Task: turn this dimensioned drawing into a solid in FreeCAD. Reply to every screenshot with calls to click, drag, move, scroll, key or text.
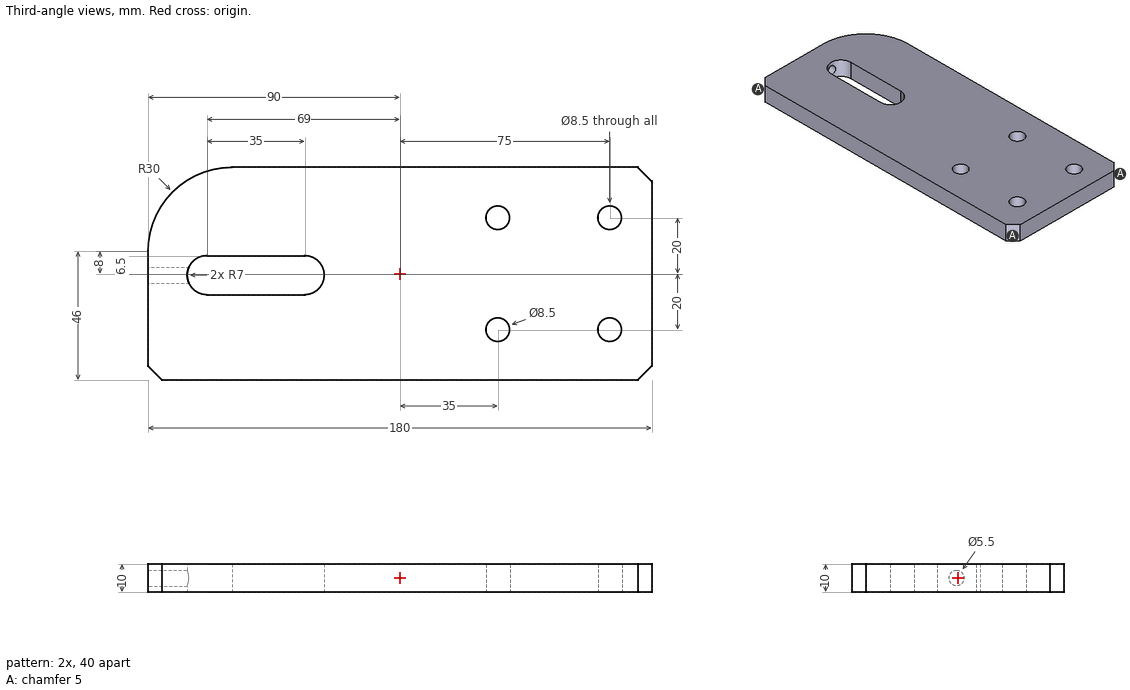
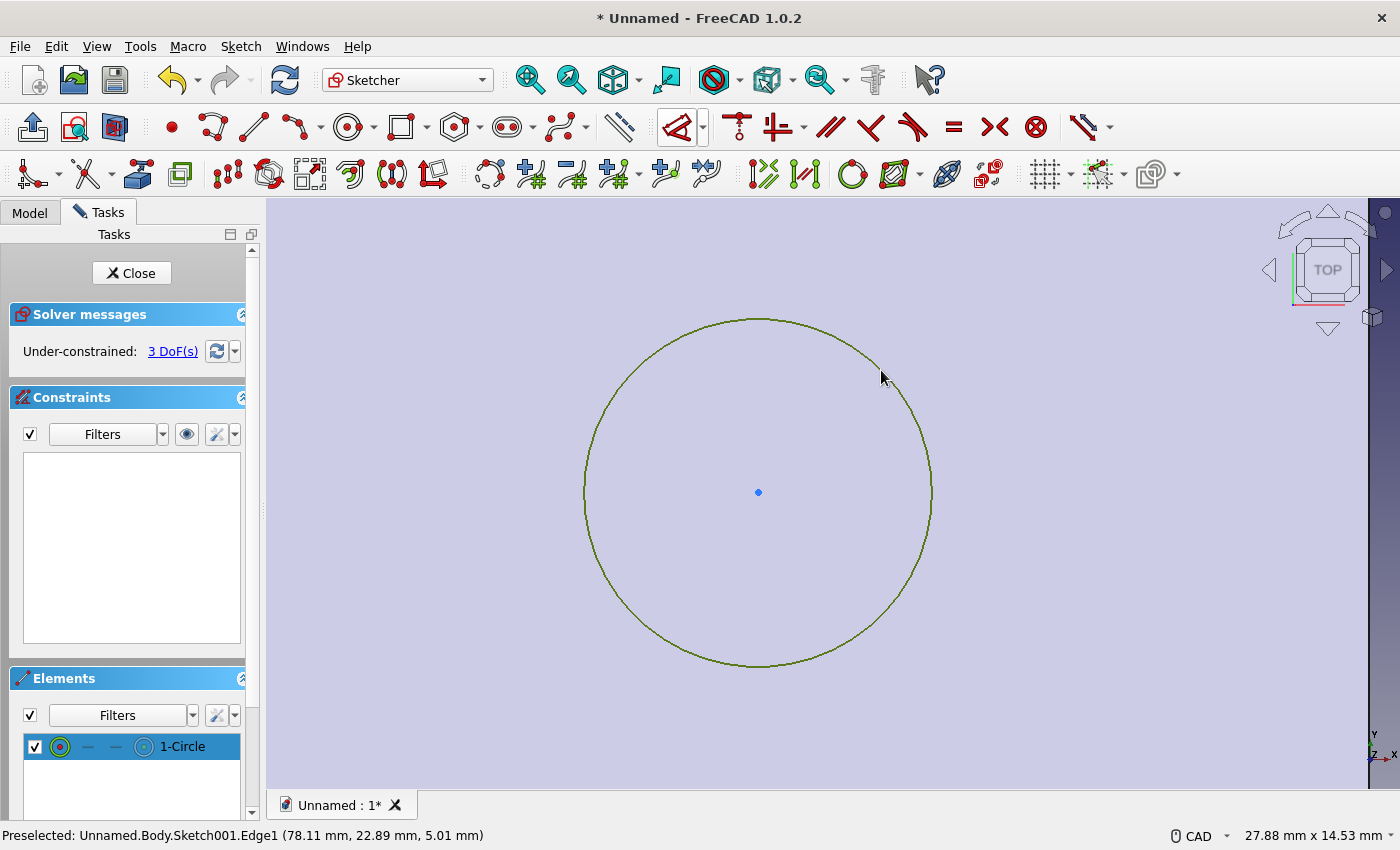
key(k)
key(o)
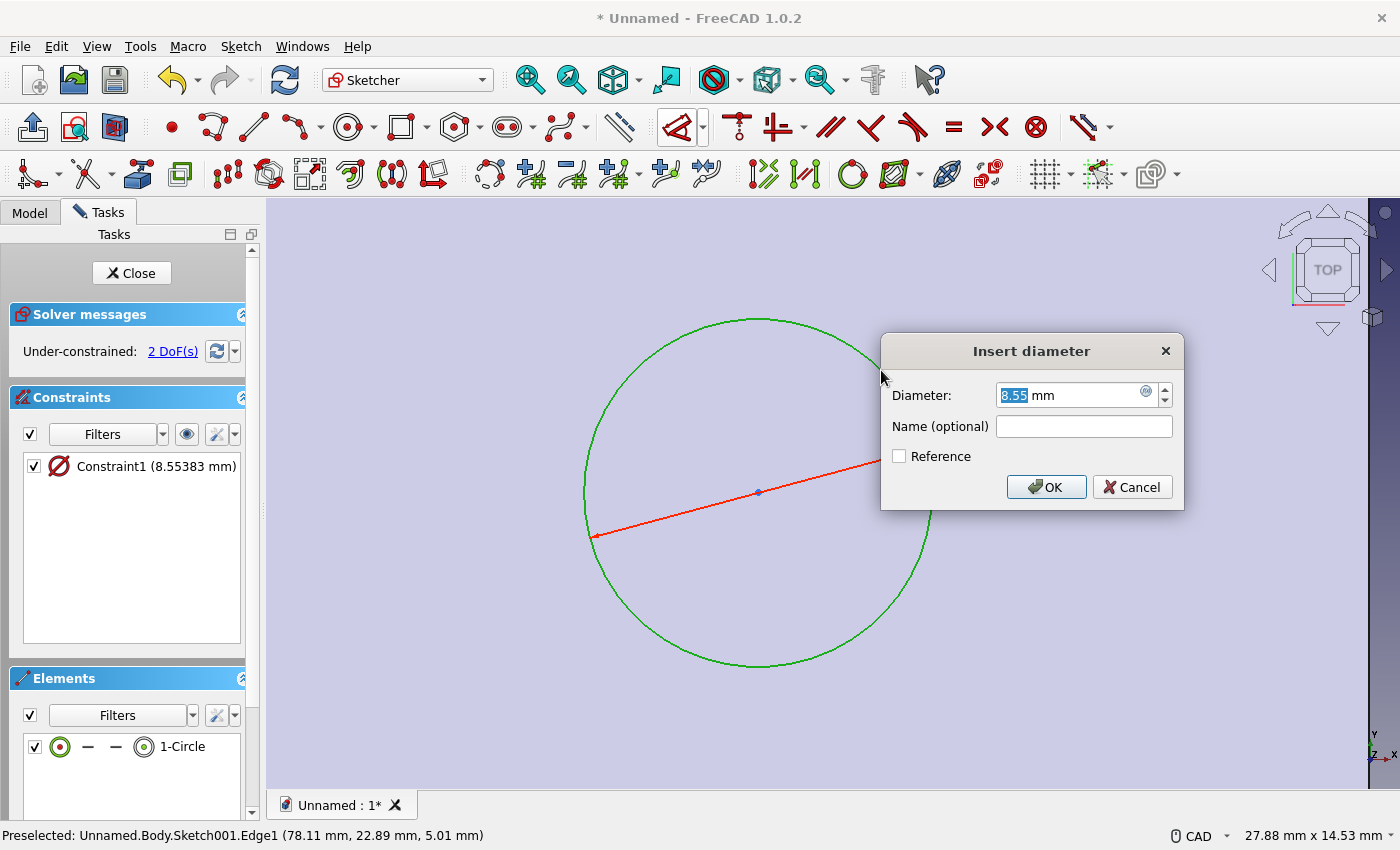
text(8.5)
key(Return)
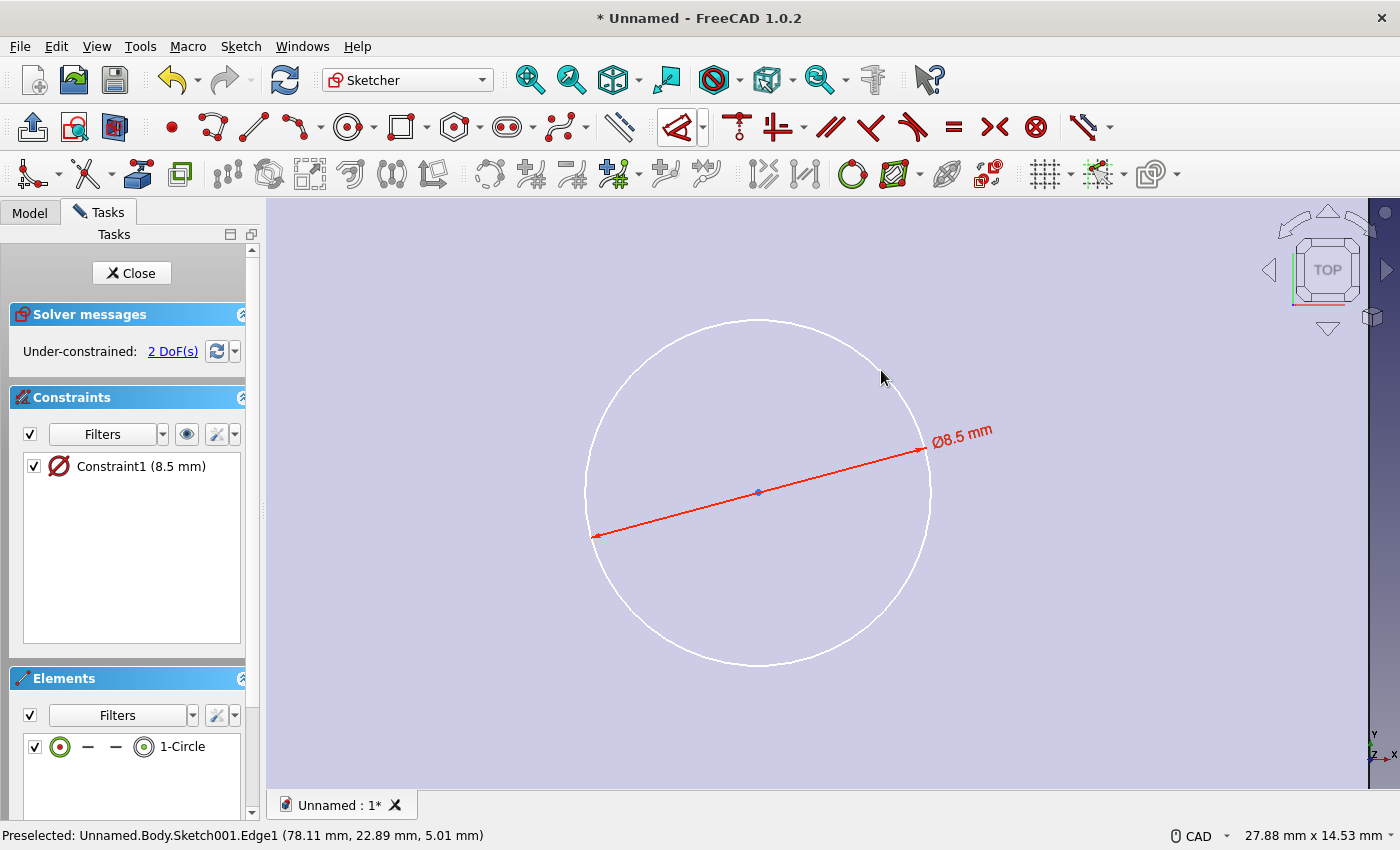
click(758, 493)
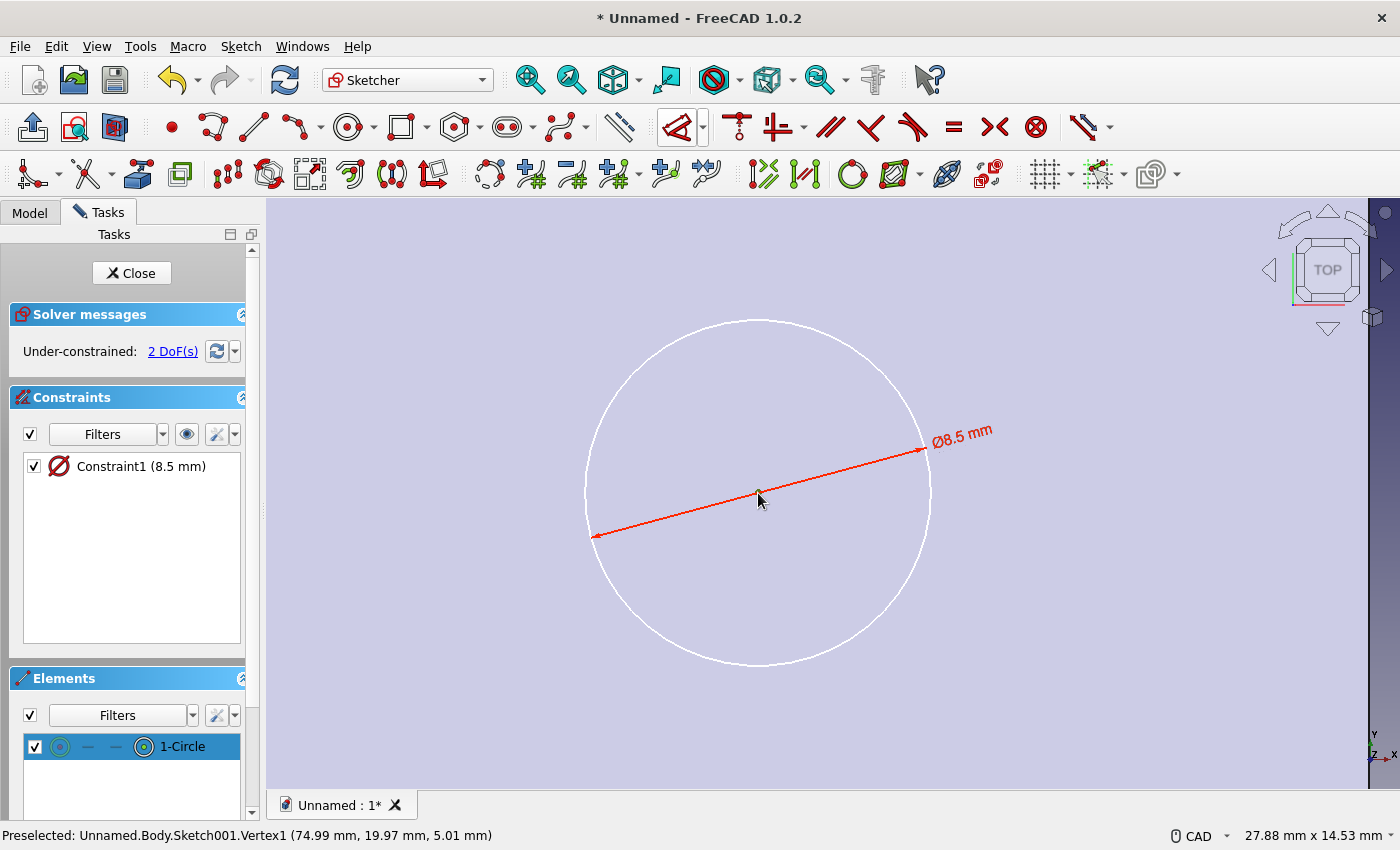
key(l)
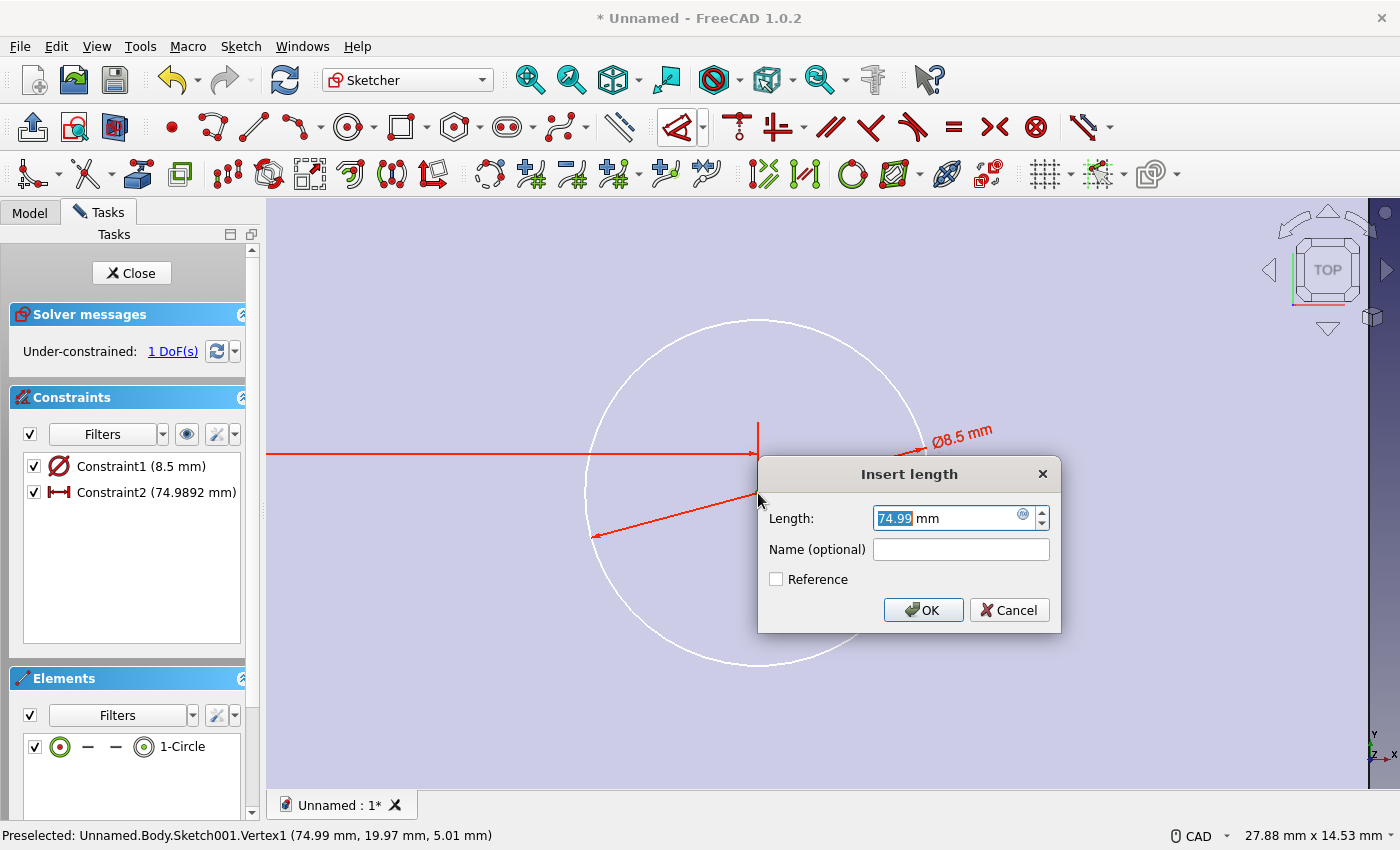
text(75)
key(Return)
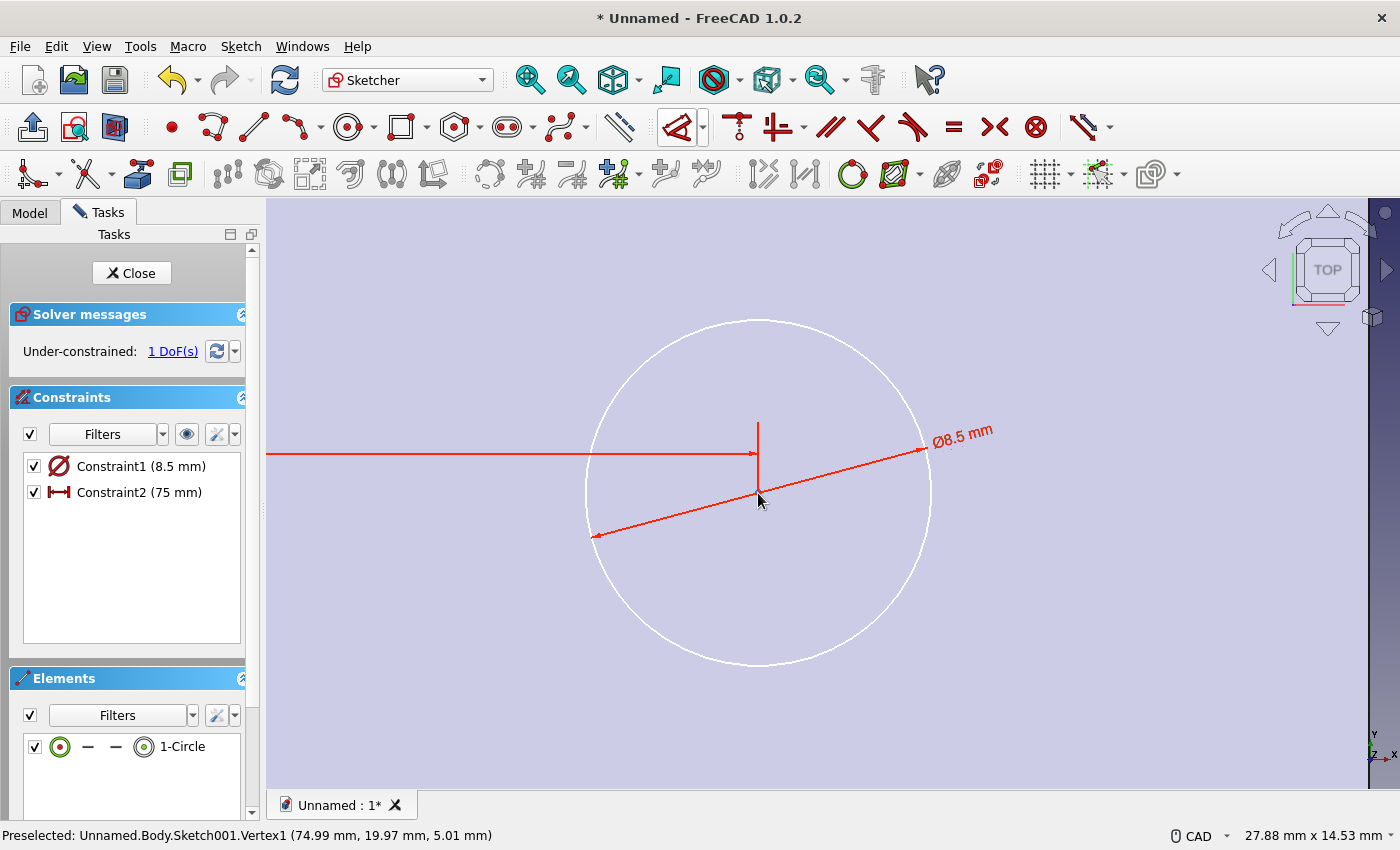
click(758, 493)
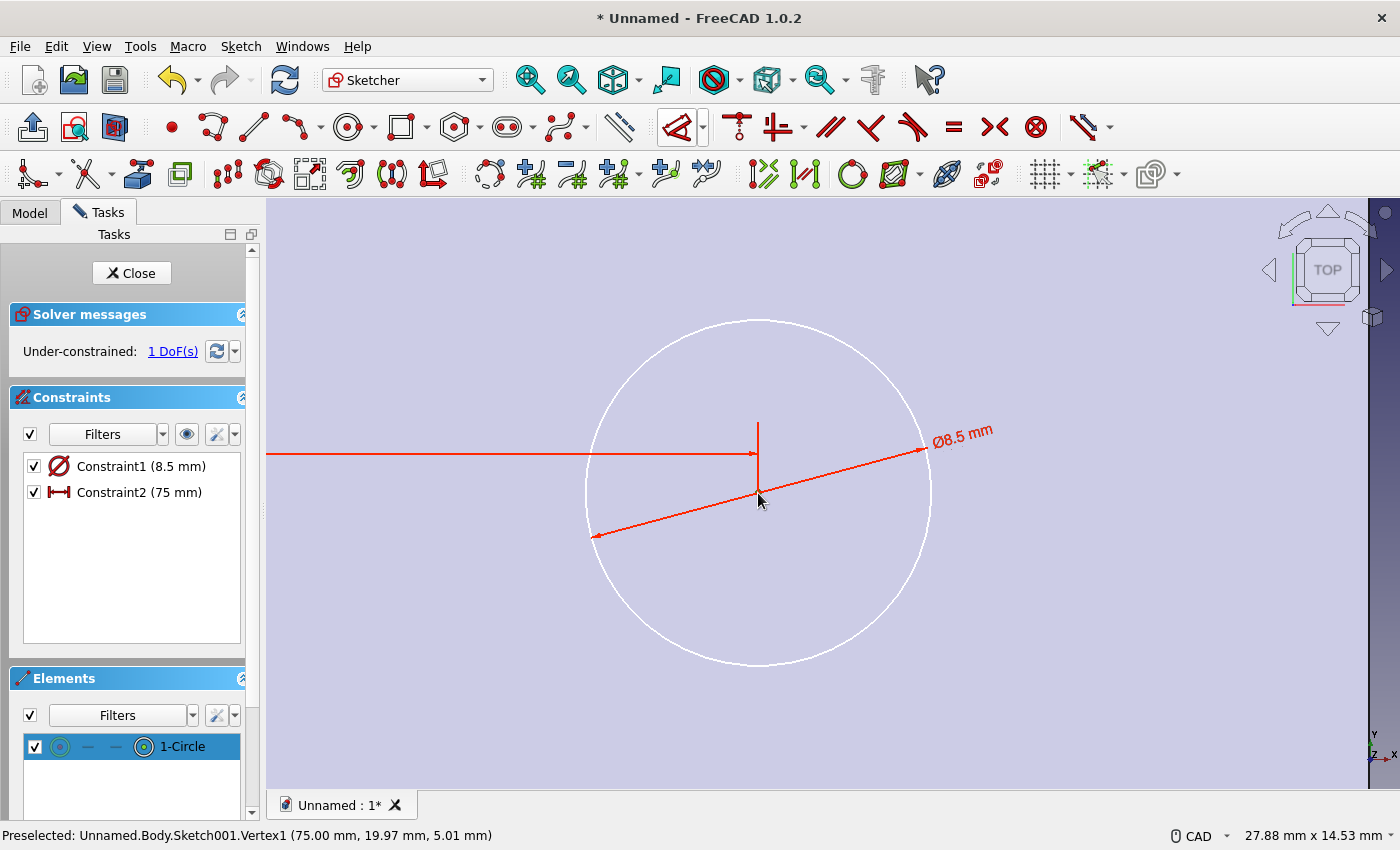
key(i)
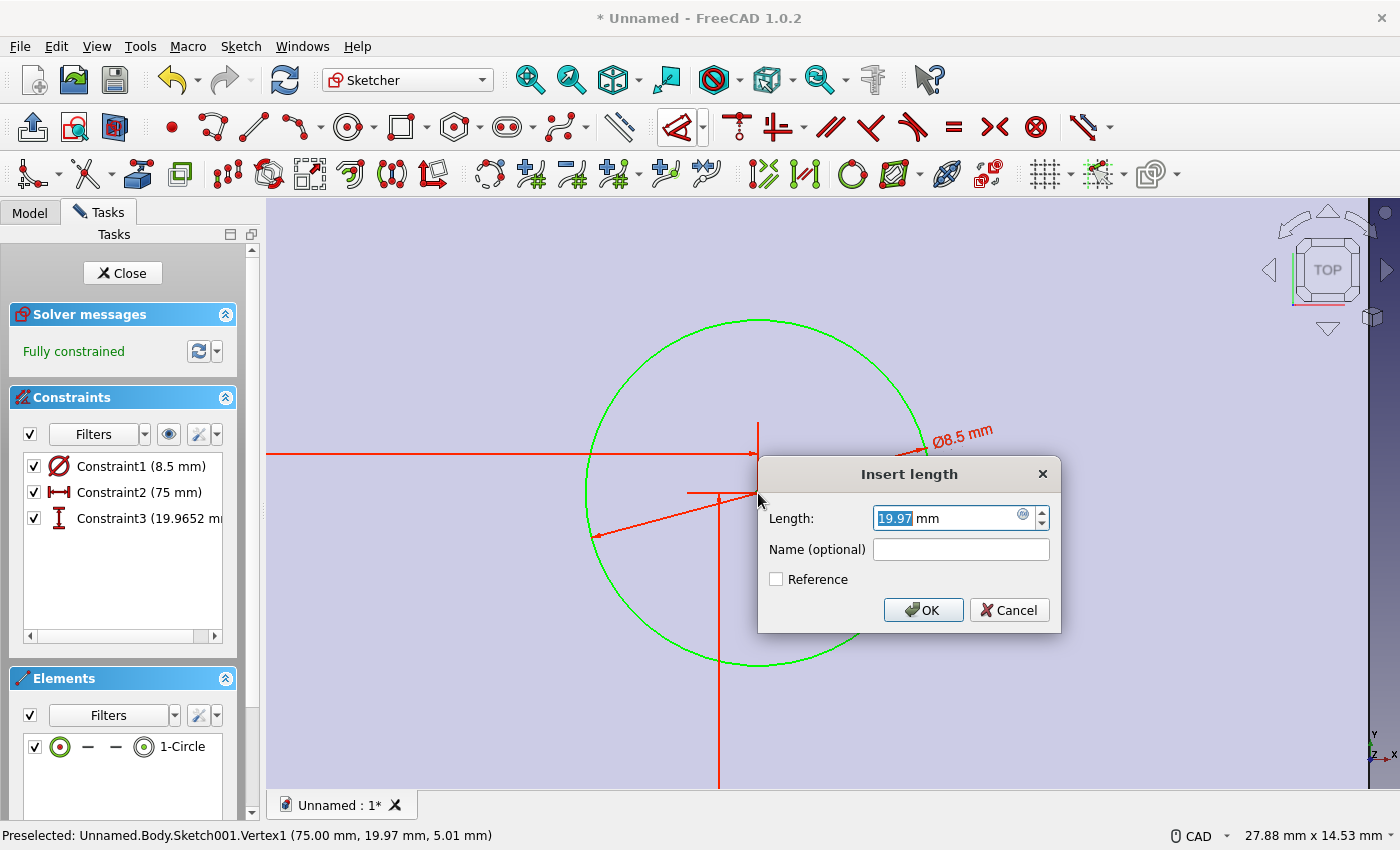
text(20)
key(Return)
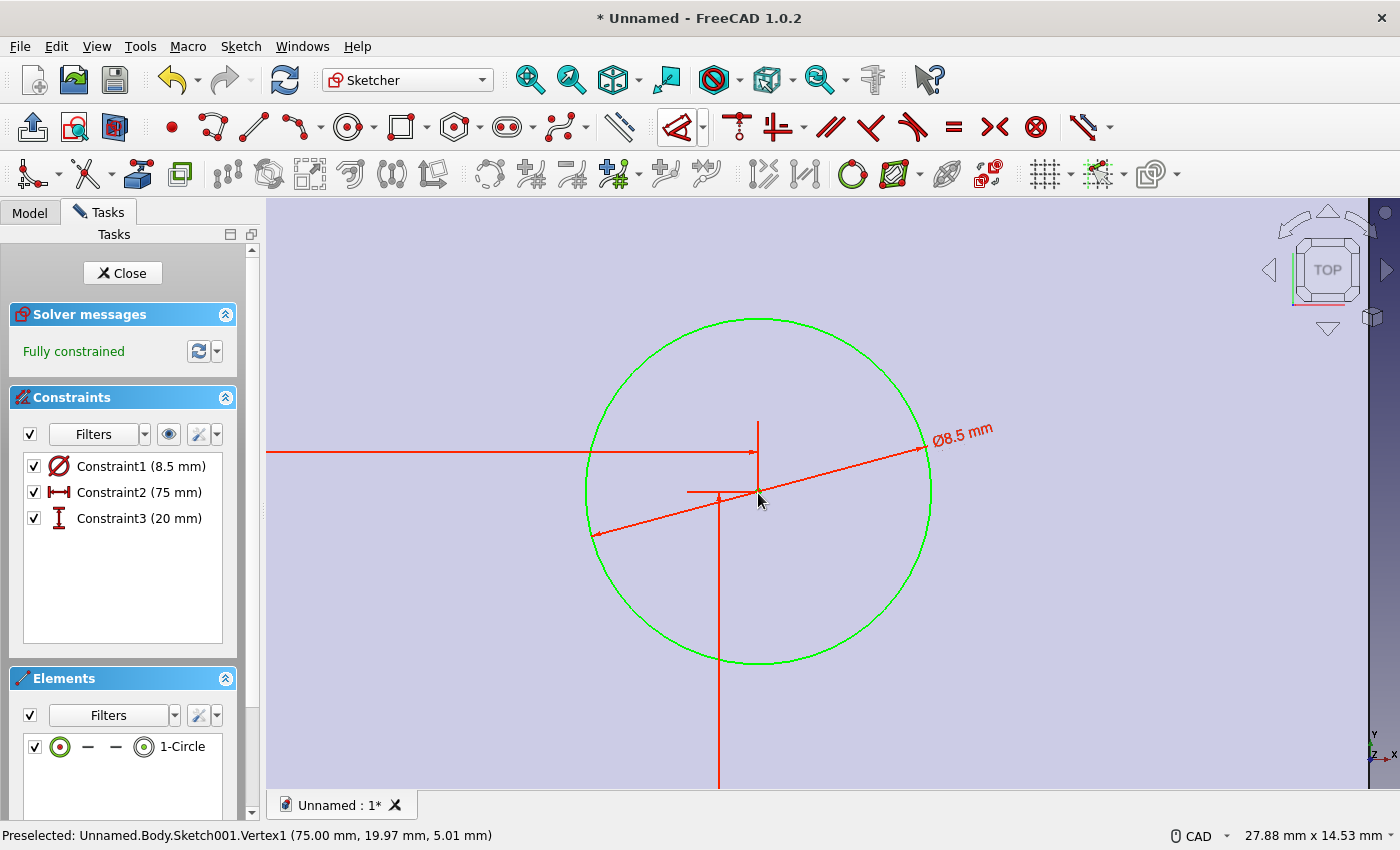
click(123, 273)